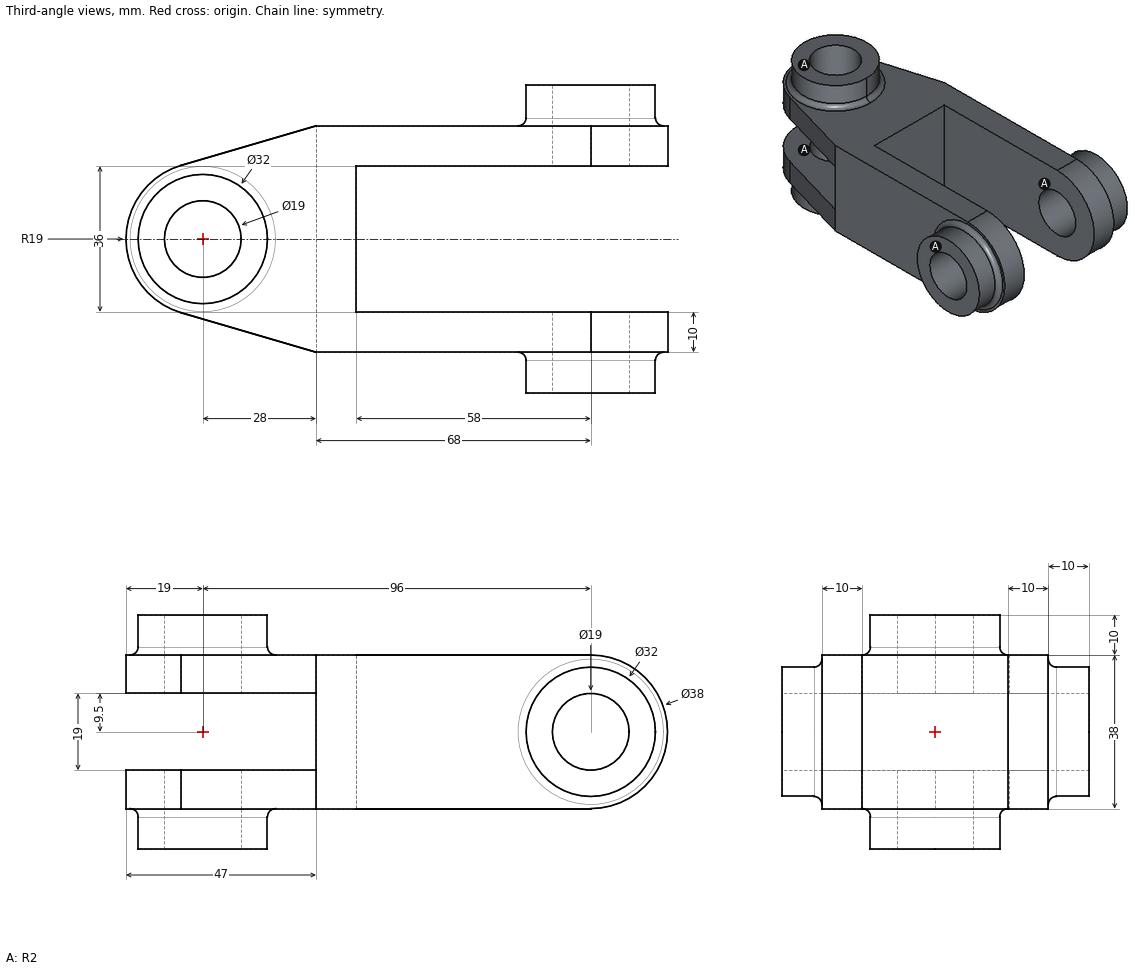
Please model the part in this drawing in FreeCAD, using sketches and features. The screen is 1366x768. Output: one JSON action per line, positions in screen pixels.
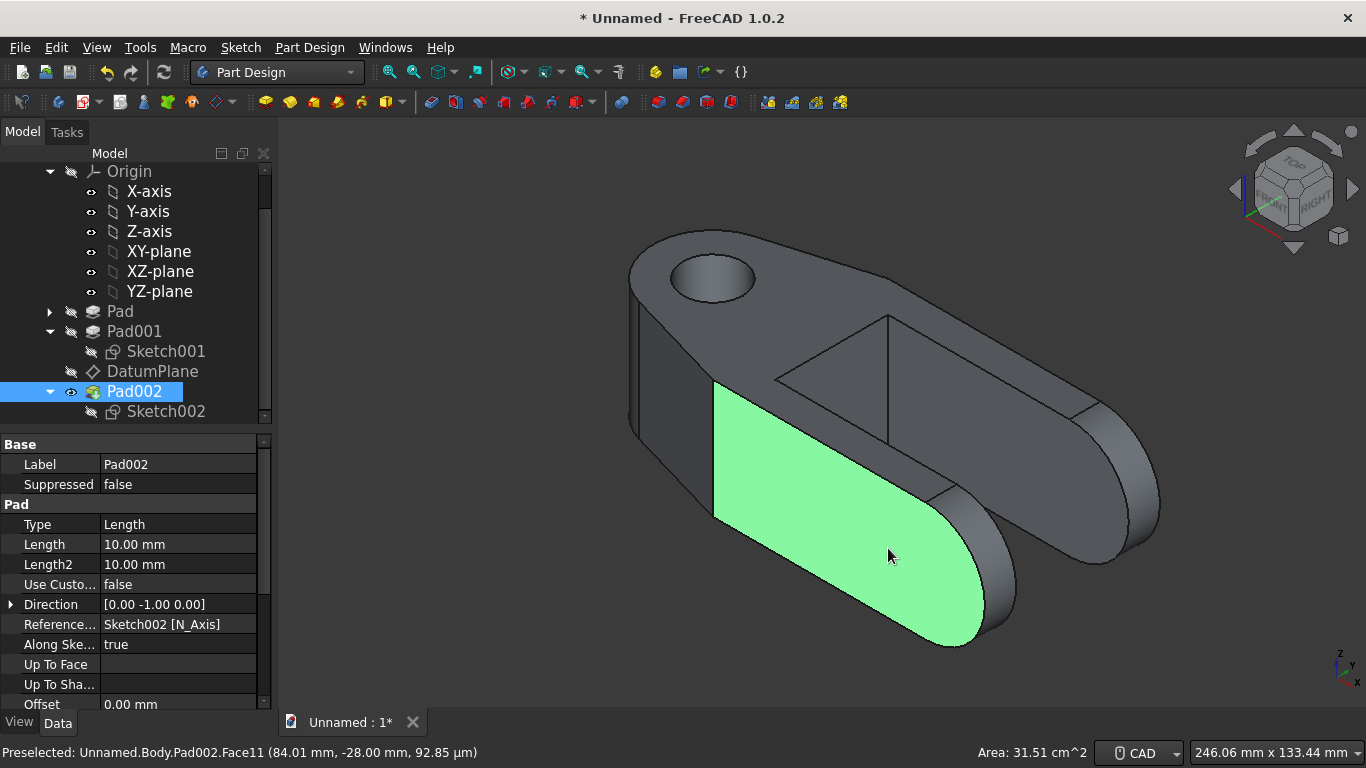
{"action": "left_click", "coordinate": [84, 102]}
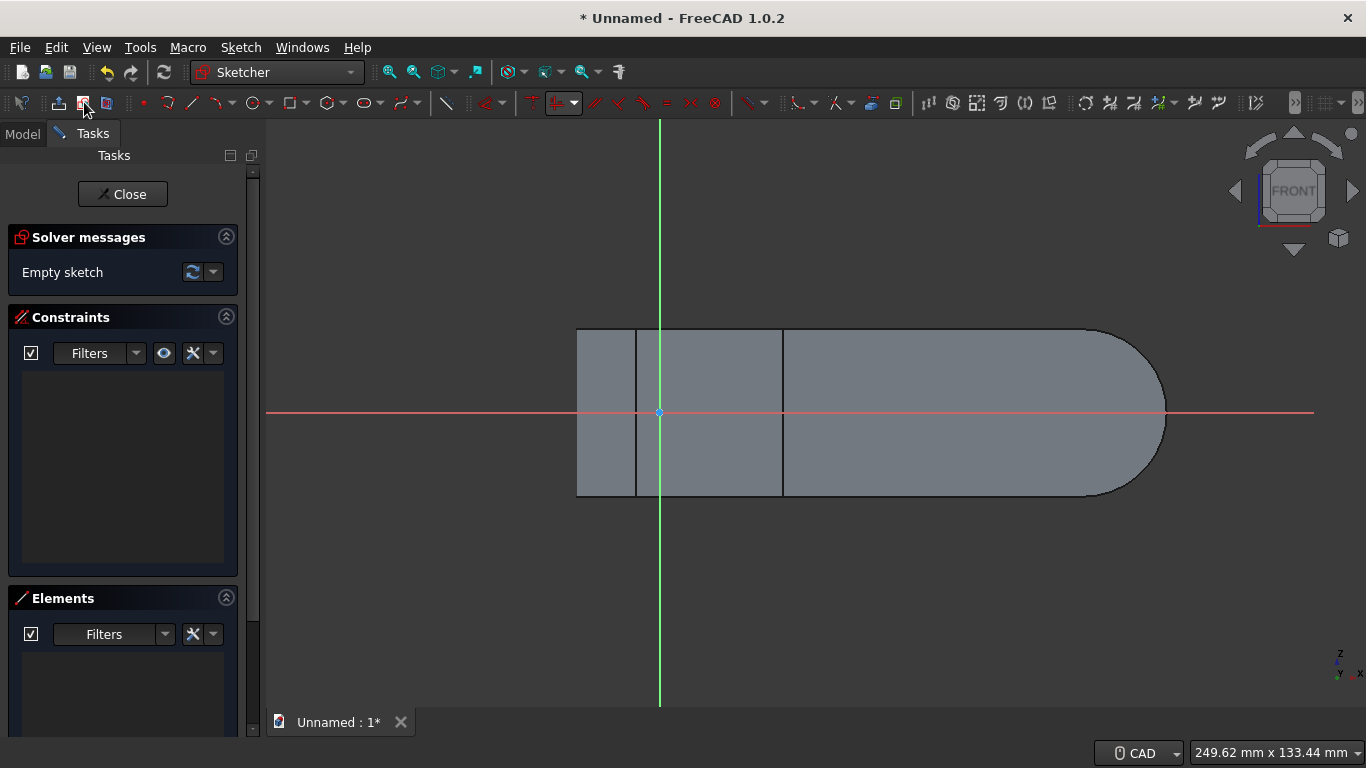
{"action": "scroll", "coordinate": [651, 413], "scroll_direction": "up", "scroll_amount": 6}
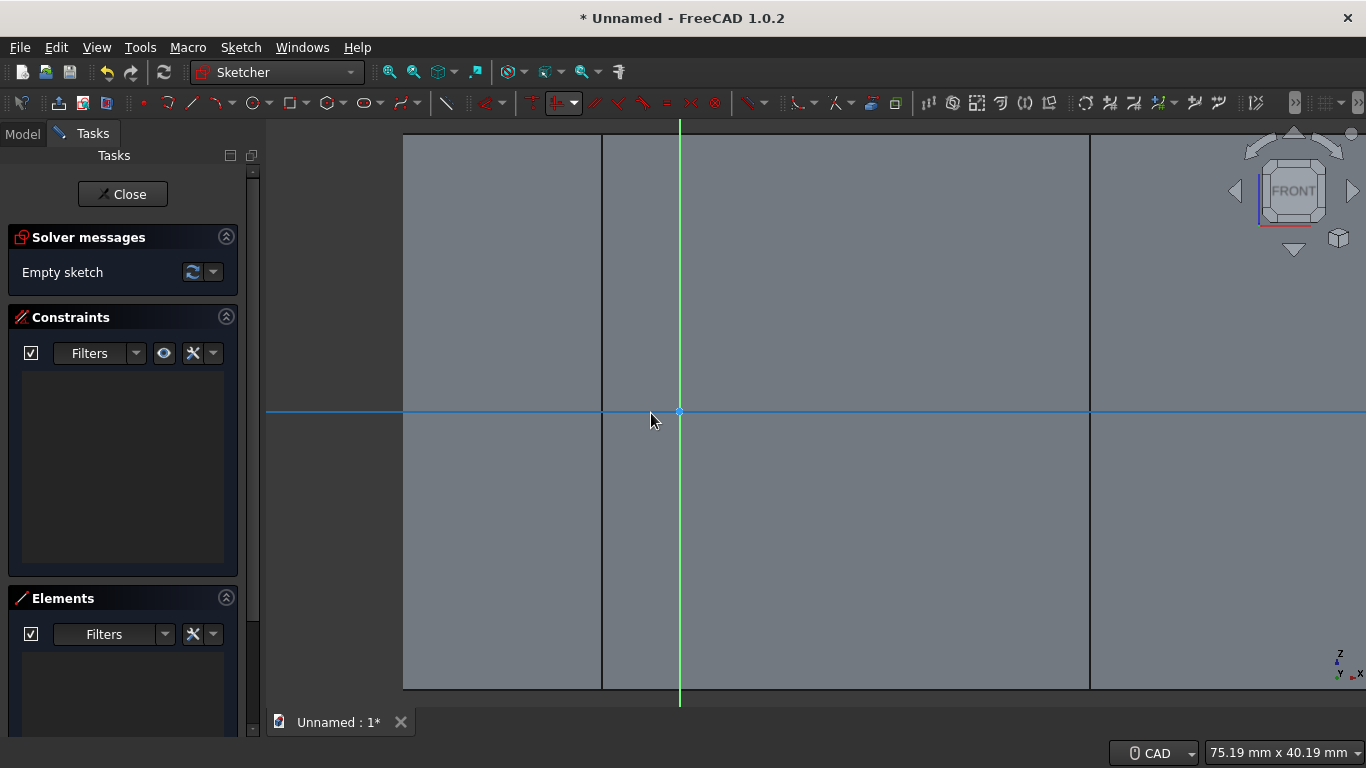
{"action": "left_click", "coordinate": [290, 104]}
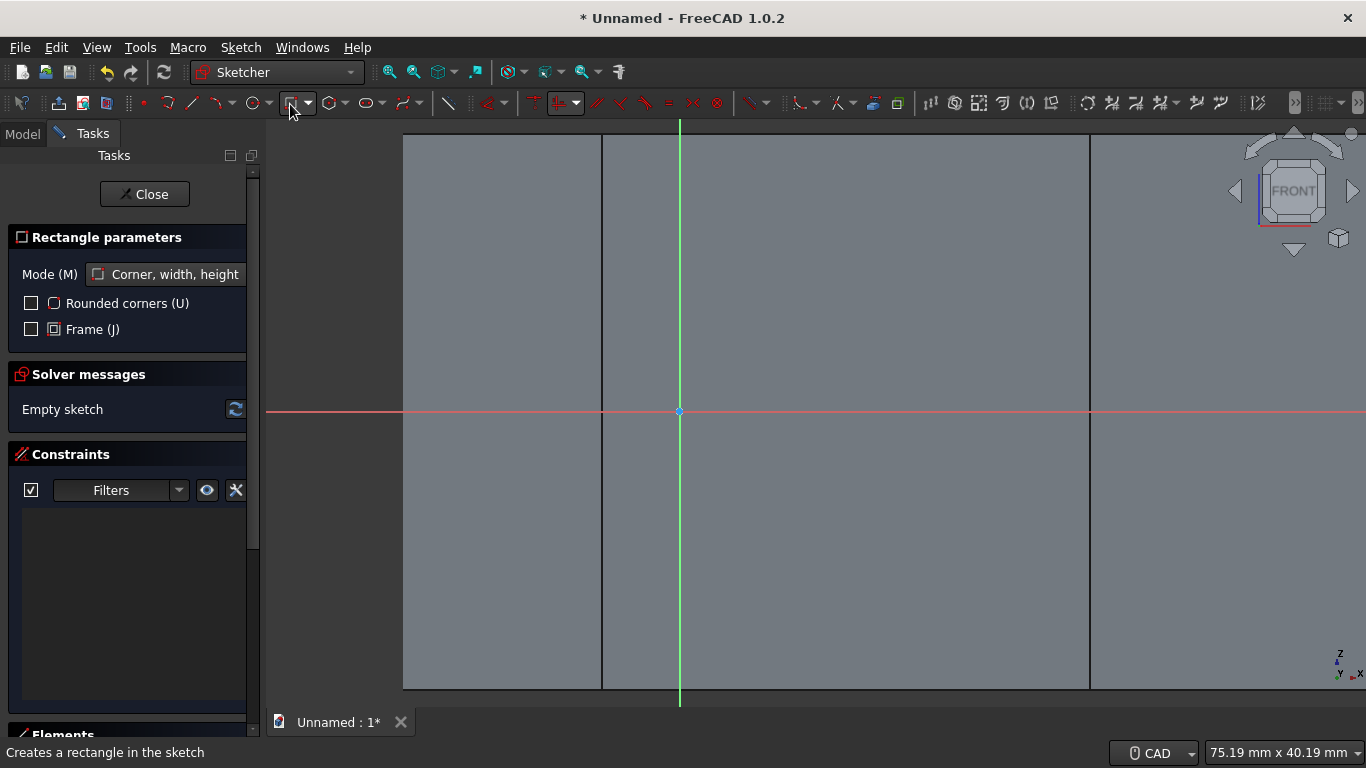
{"action": "left_click", "coordinate": [402, 273]}
{"action": "left_click", "coordinate": [1090, 551]}
{"action": "key", "text": "Escape"}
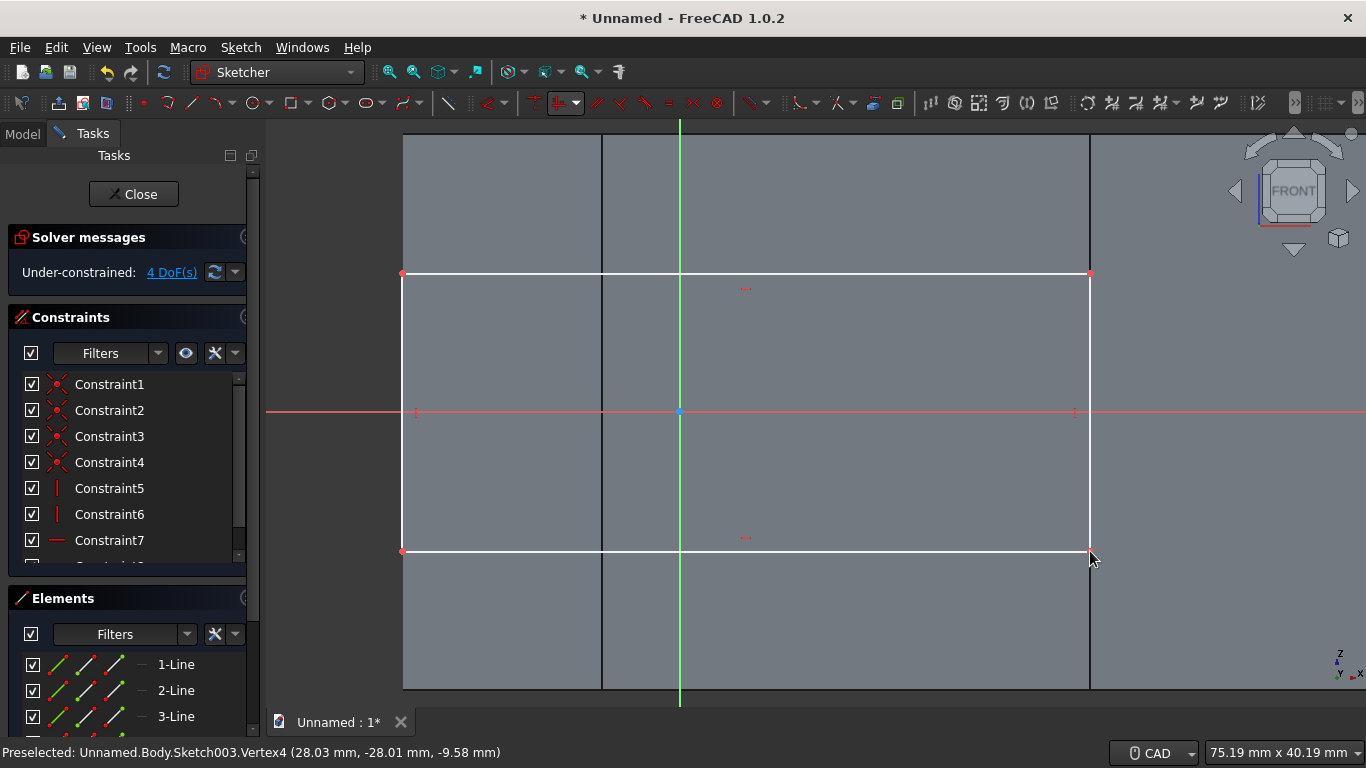
{"action": "left_click", "coordinate": [488, 104]}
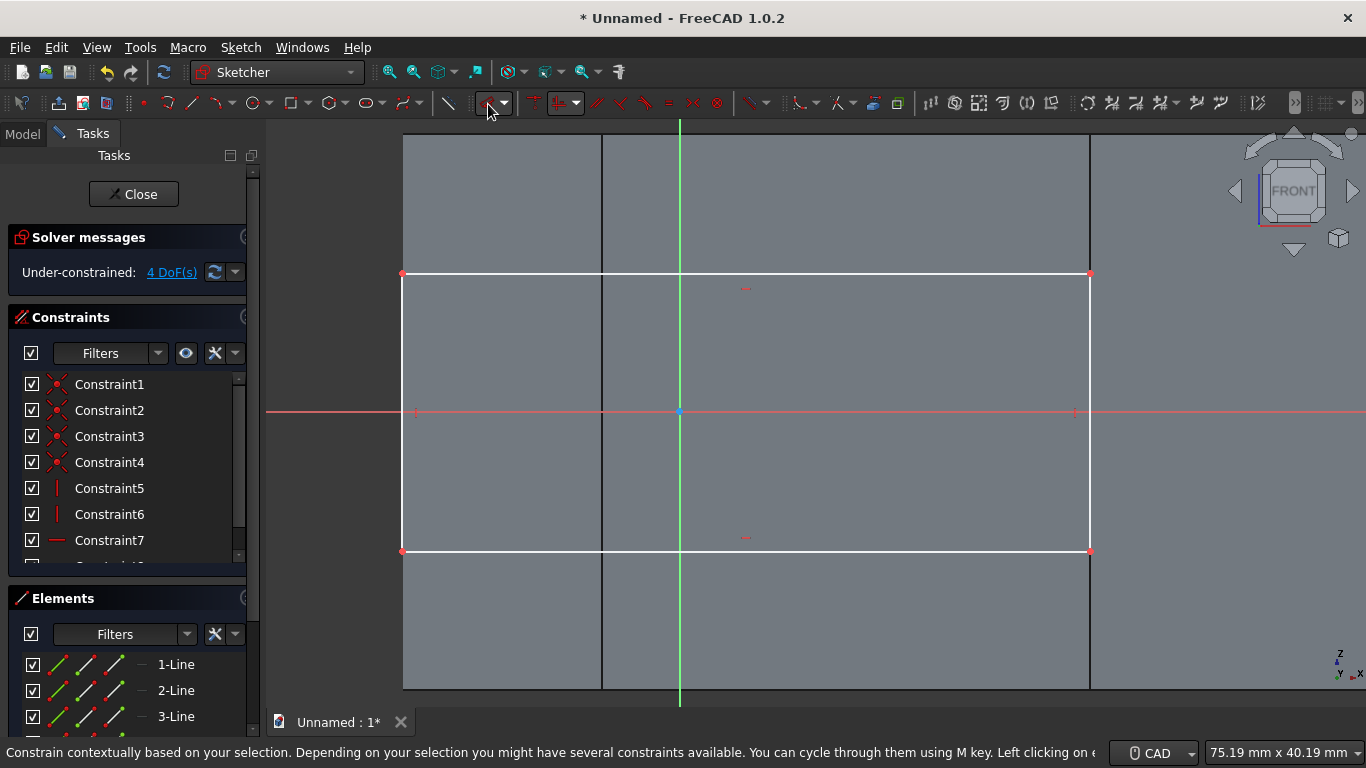
{"action": "left_click", "coordinate": [402, 357]}
{"action": "left_click", "coordinate": [368, 349]}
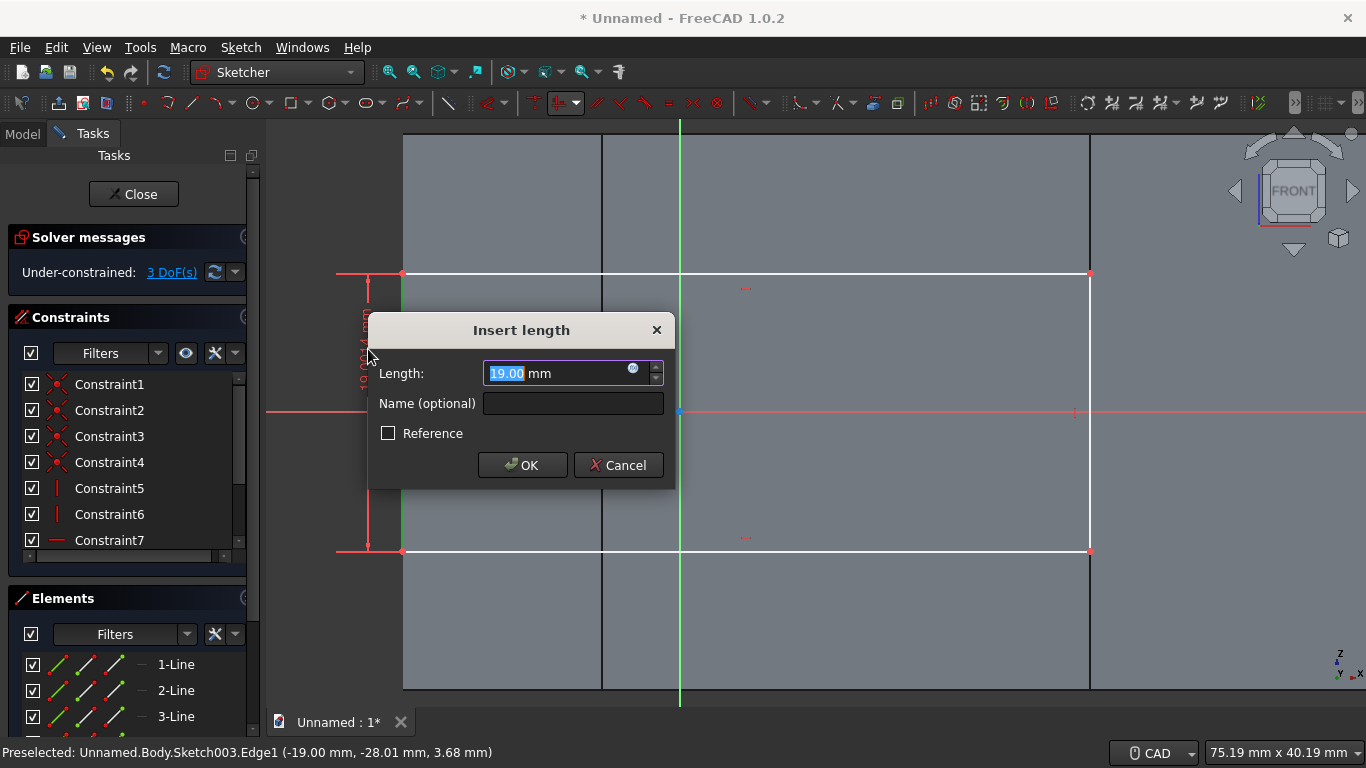
{"action": "type", "text": "19"}
{"action": "key", "text": "Return"}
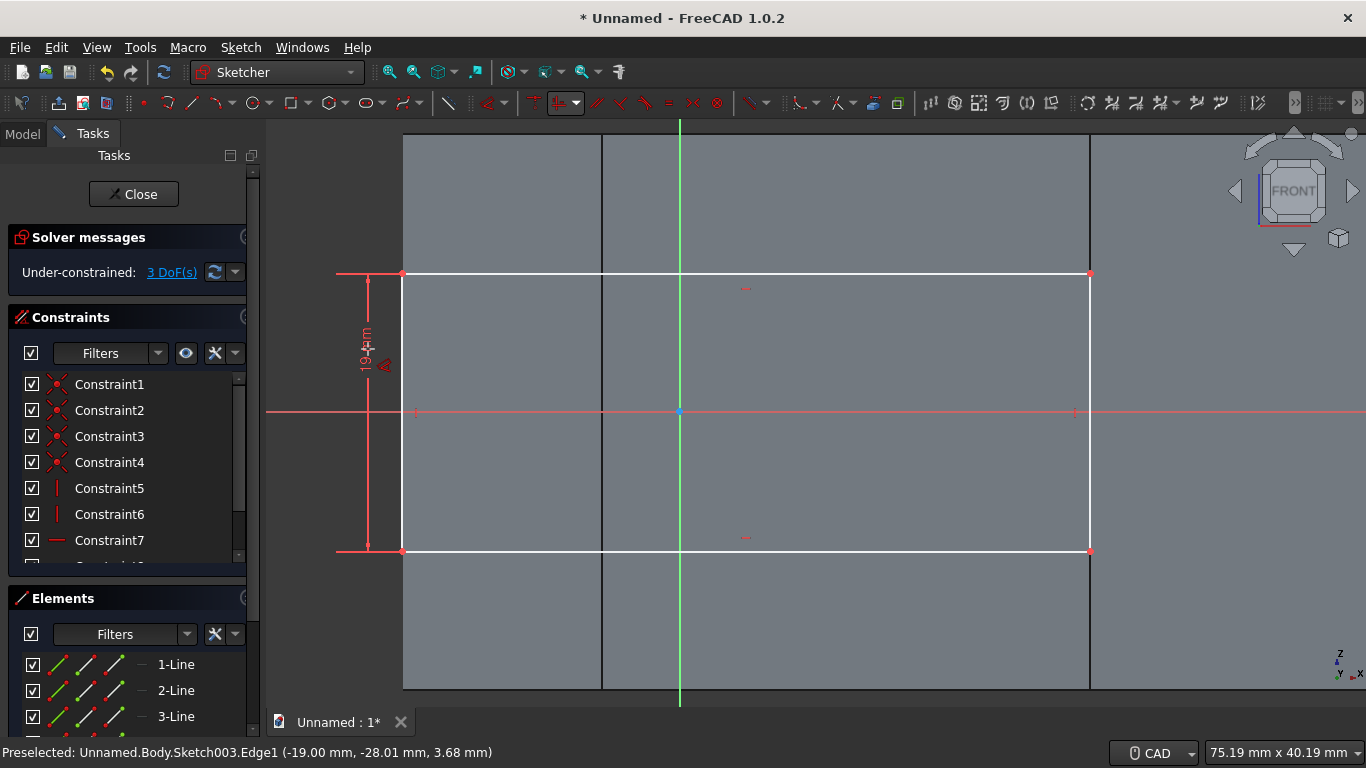
{"action": "left_click", "coordinate": [608, 552]}
{"action": "left_click", "coordinate": [746, 586]}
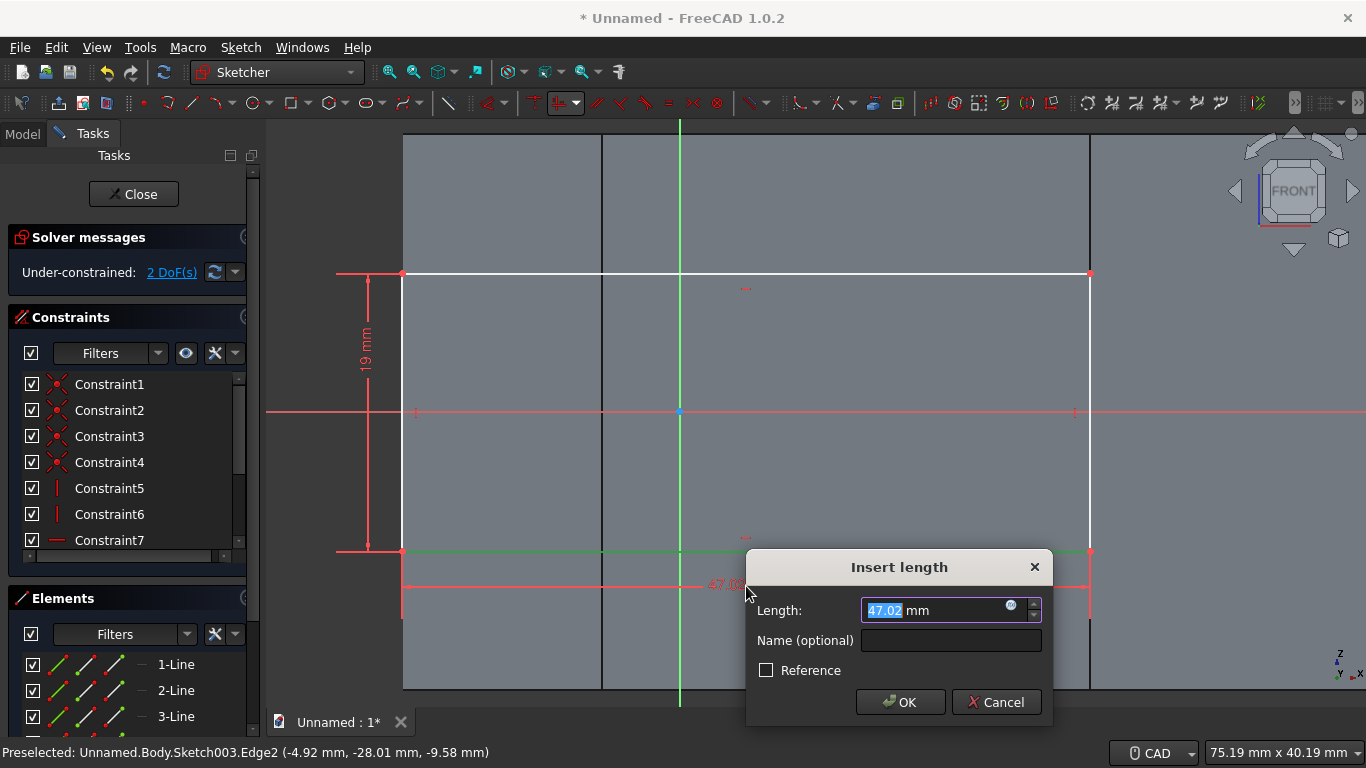
{"action": "type", "text": "47"}
{"action": "key", "text": "Return"}